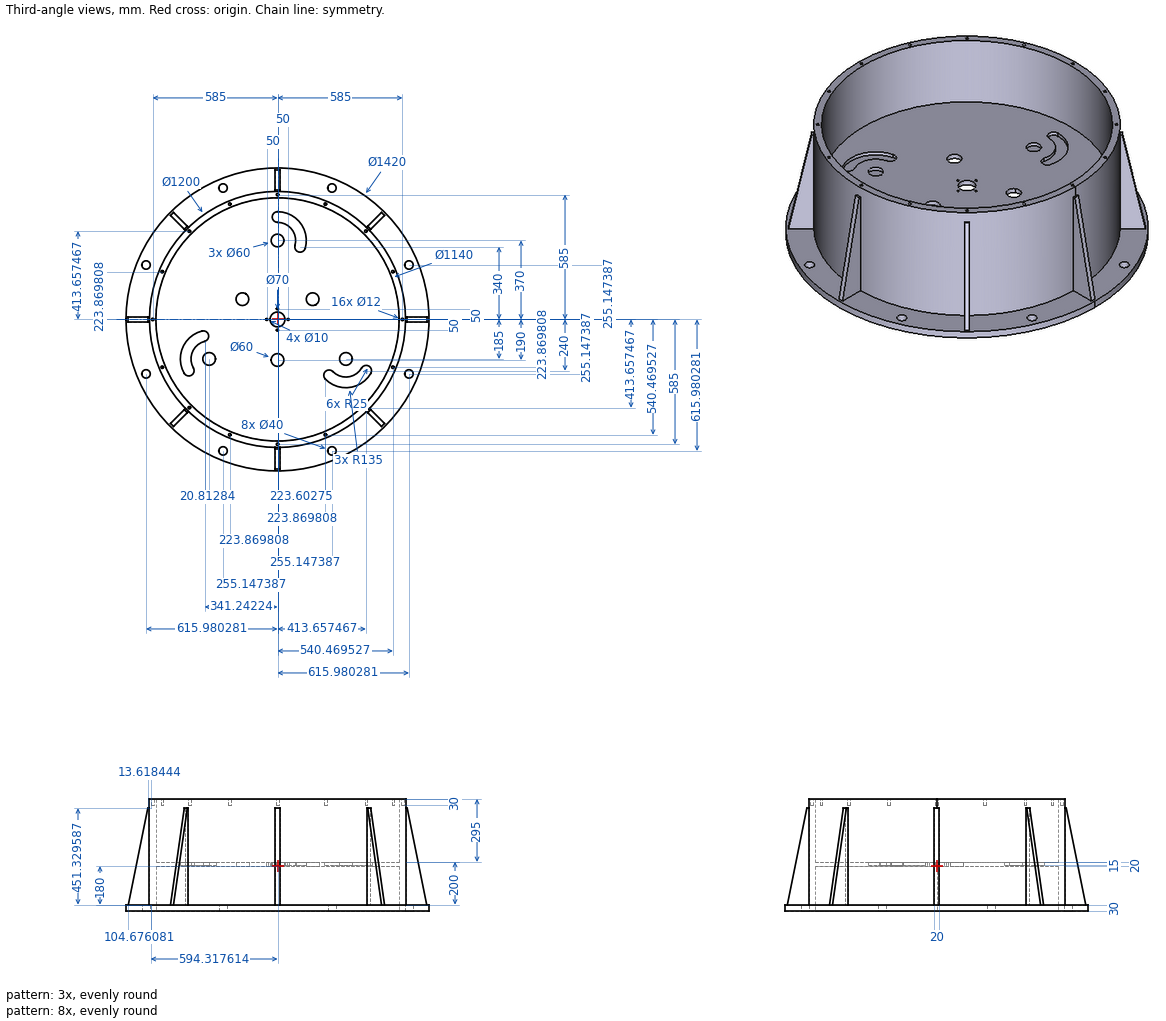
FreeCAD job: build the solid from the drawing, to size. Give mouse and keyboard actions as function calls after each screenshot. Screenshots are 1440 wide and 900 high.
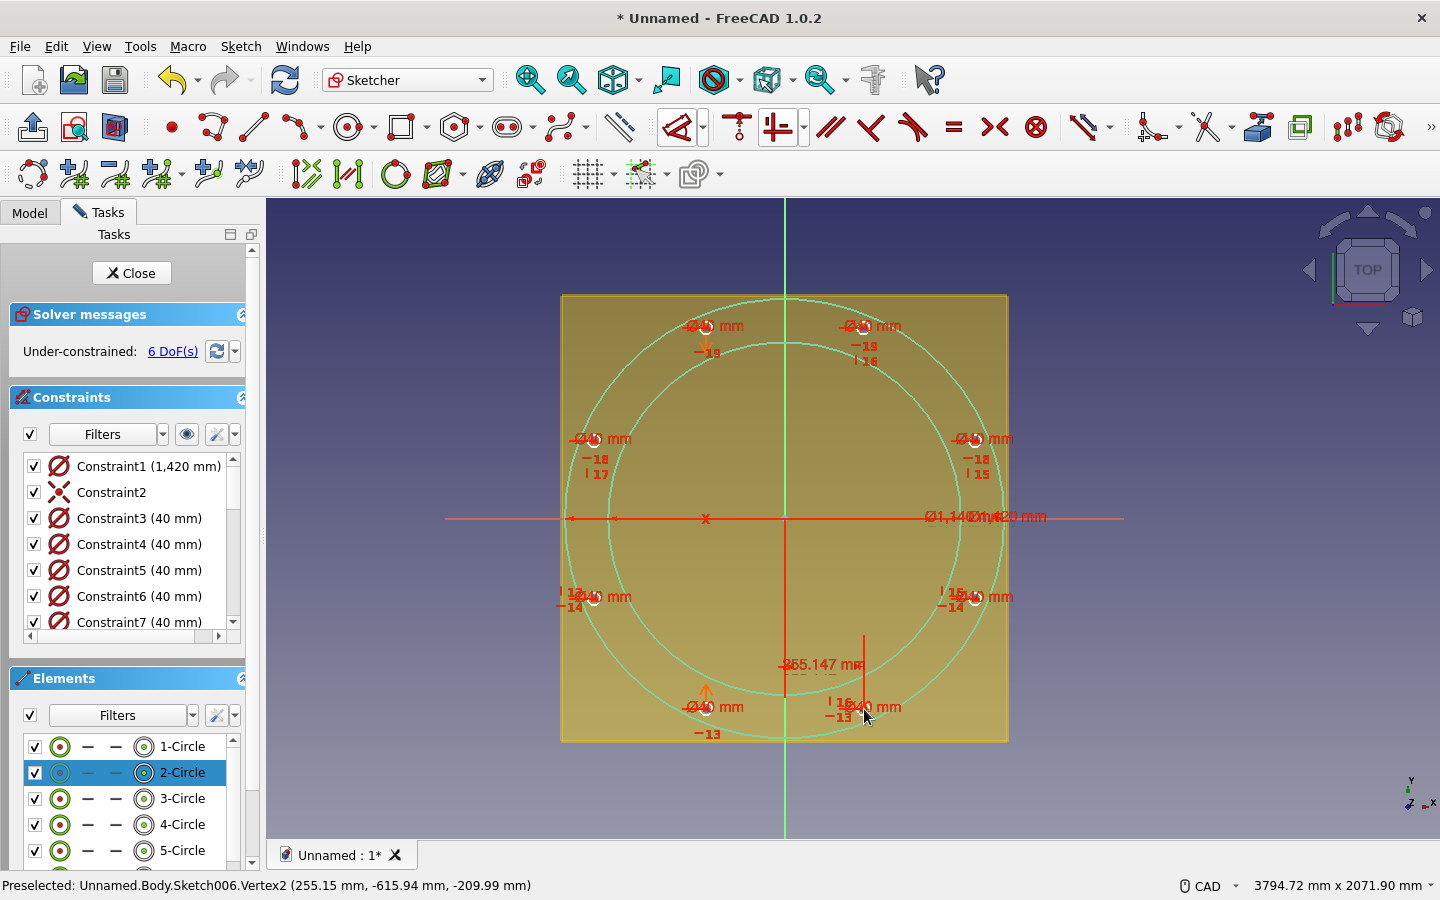
key(i)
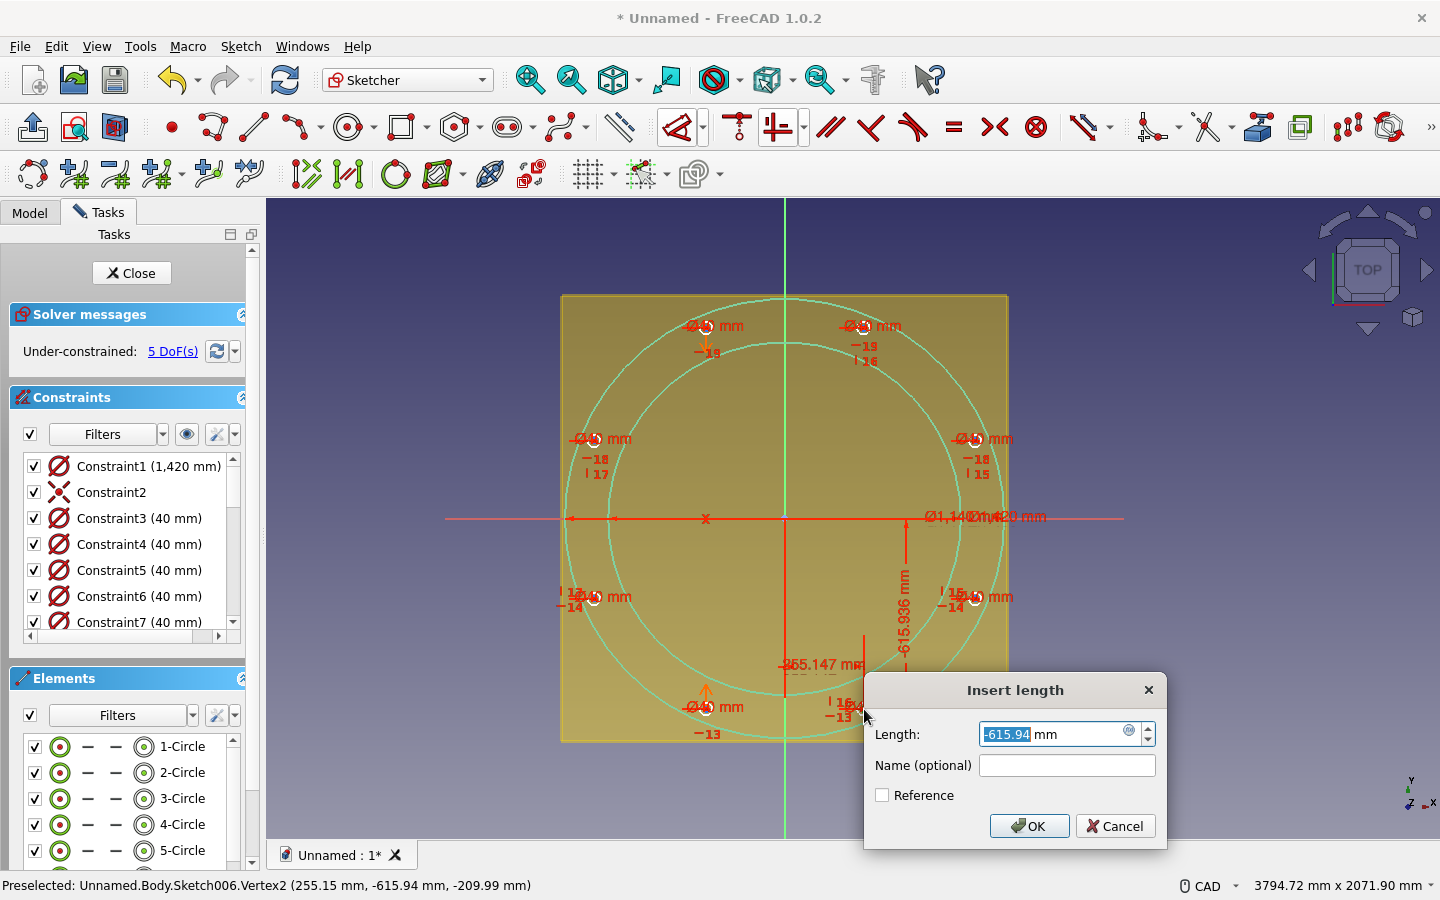
text(-615.980281)
key(Return)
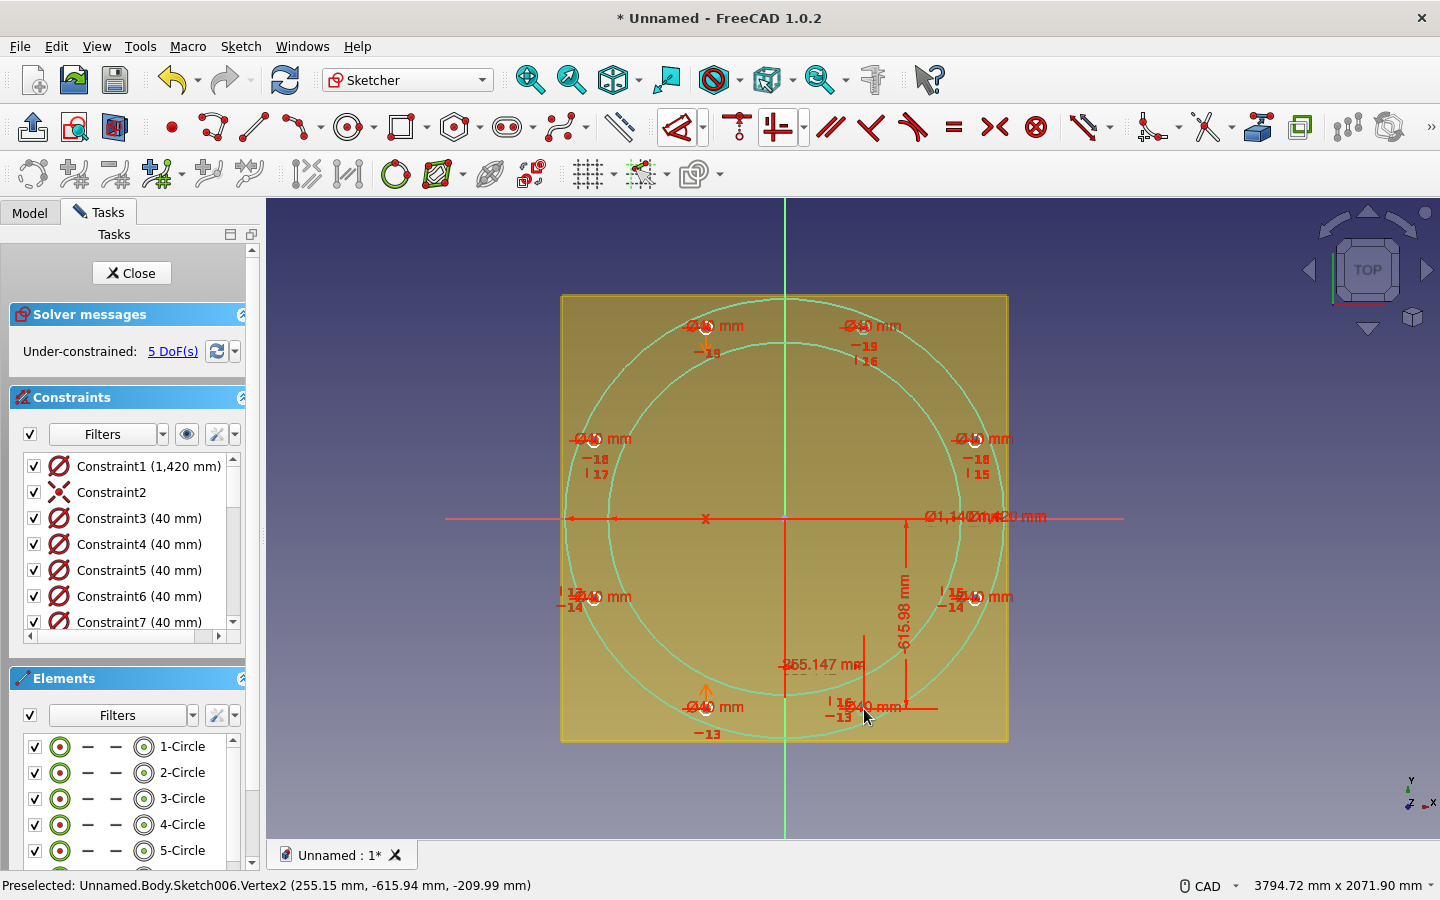
click(975, 599)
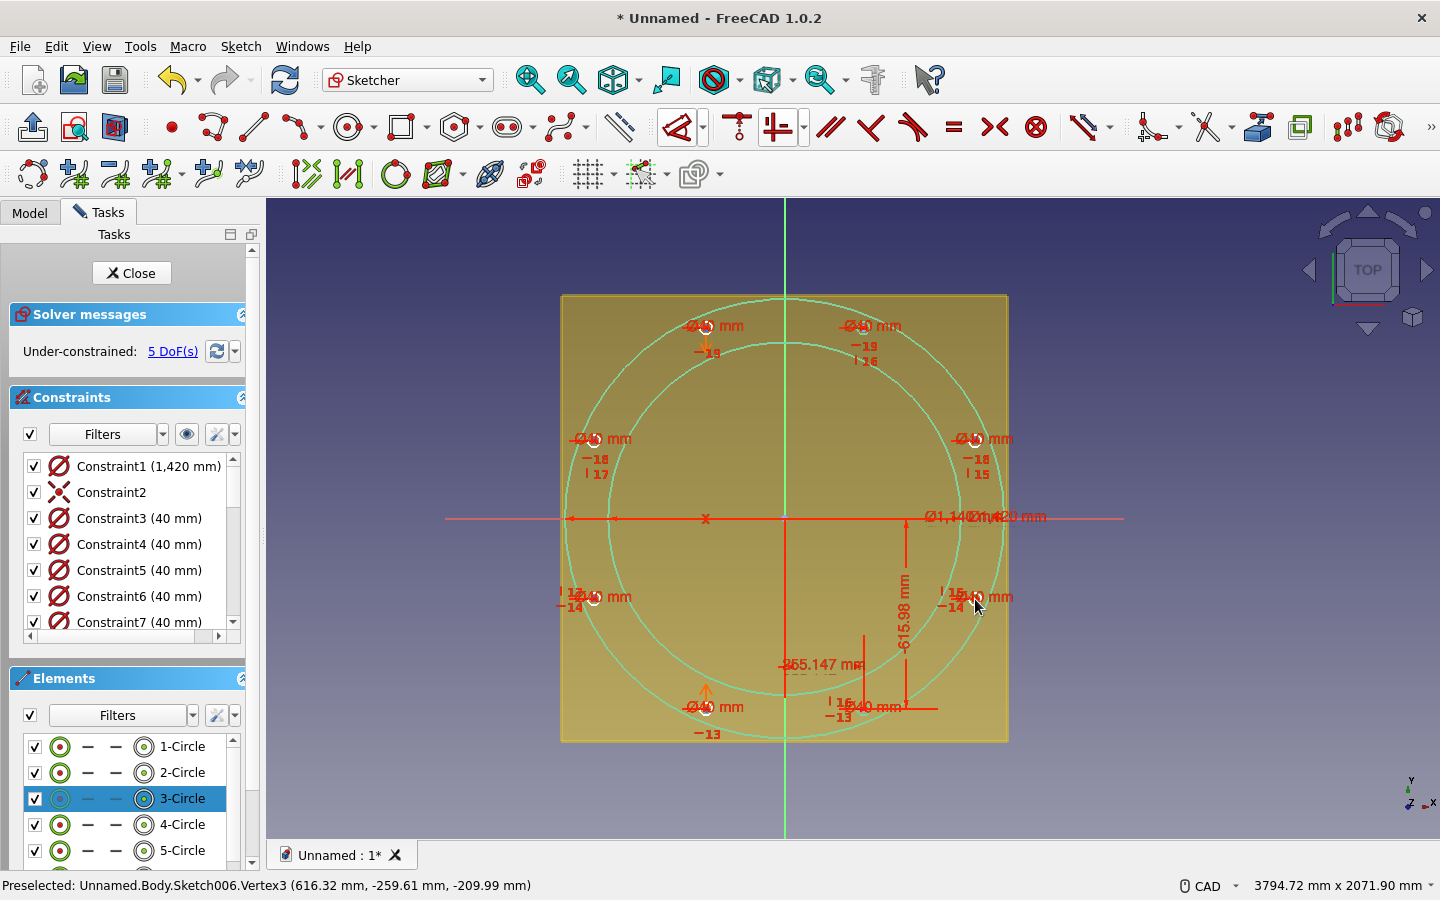
click(702, 128)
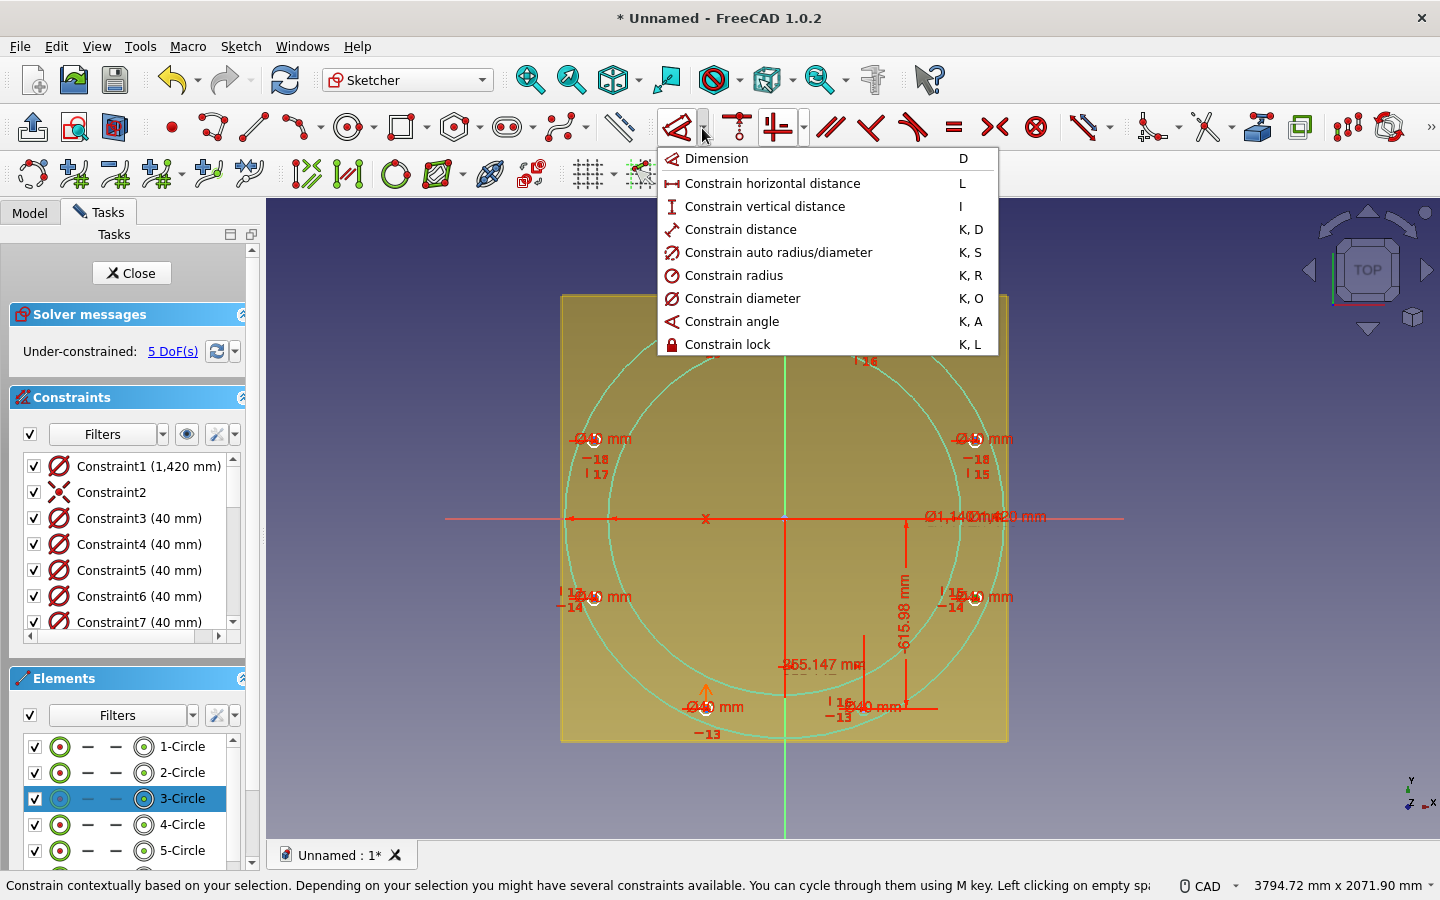
click(828, 184)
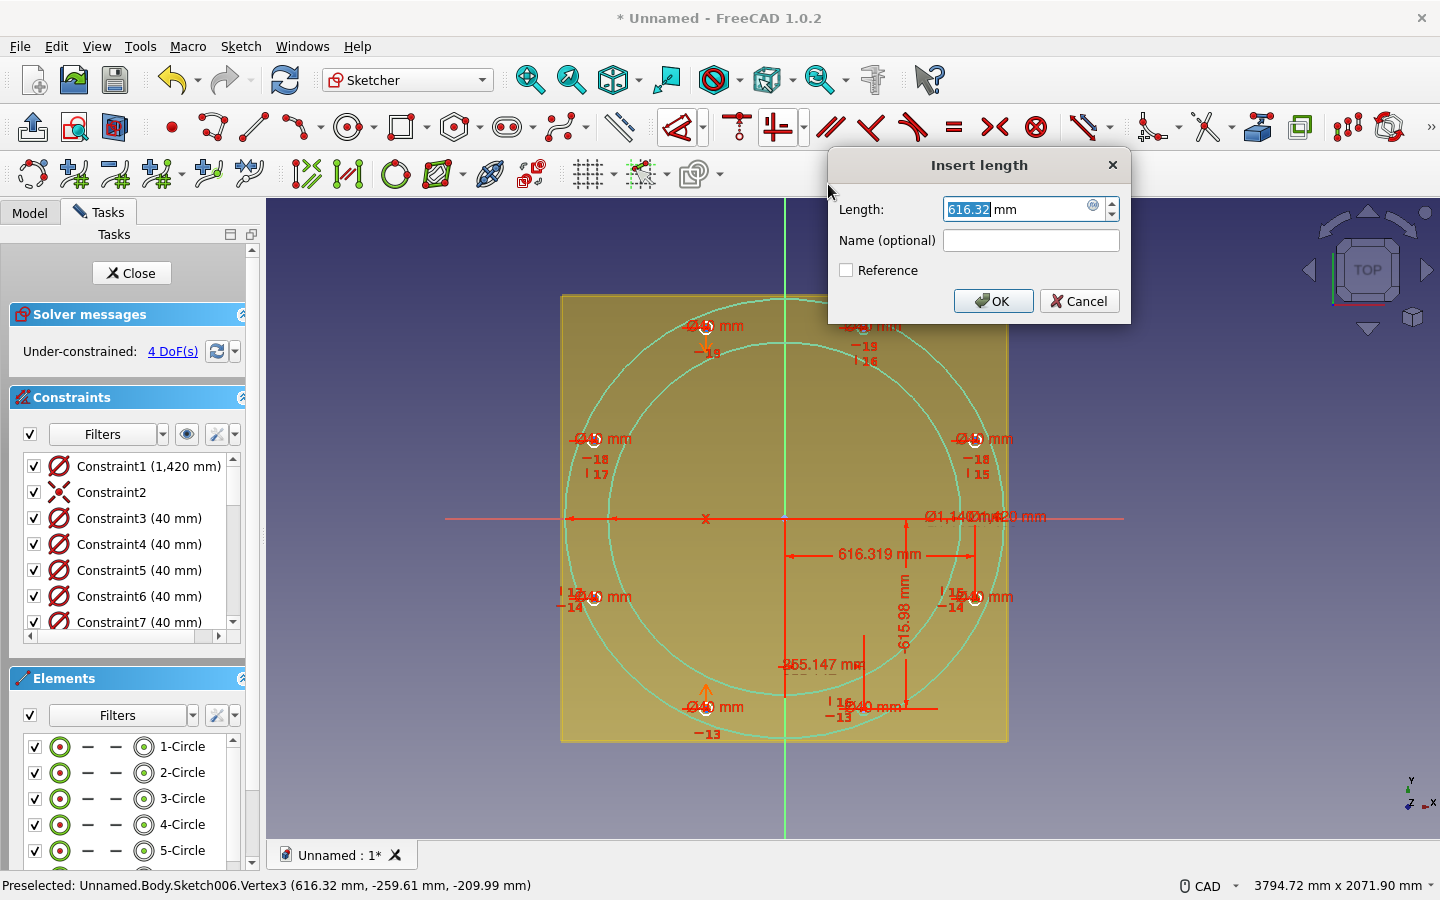
text(615.980281)
key(Return)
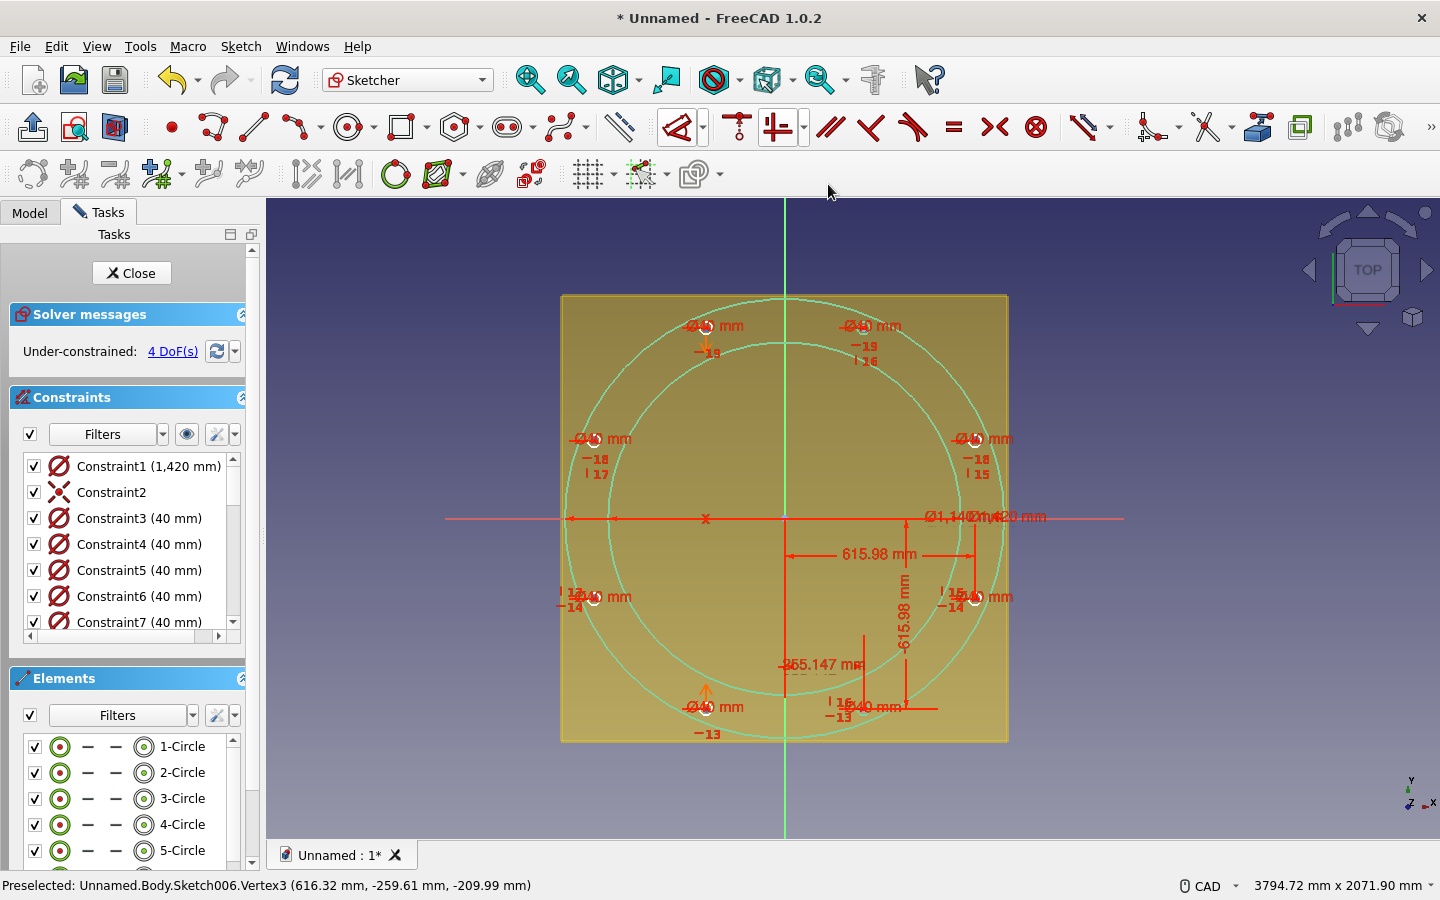
click(975, 599)